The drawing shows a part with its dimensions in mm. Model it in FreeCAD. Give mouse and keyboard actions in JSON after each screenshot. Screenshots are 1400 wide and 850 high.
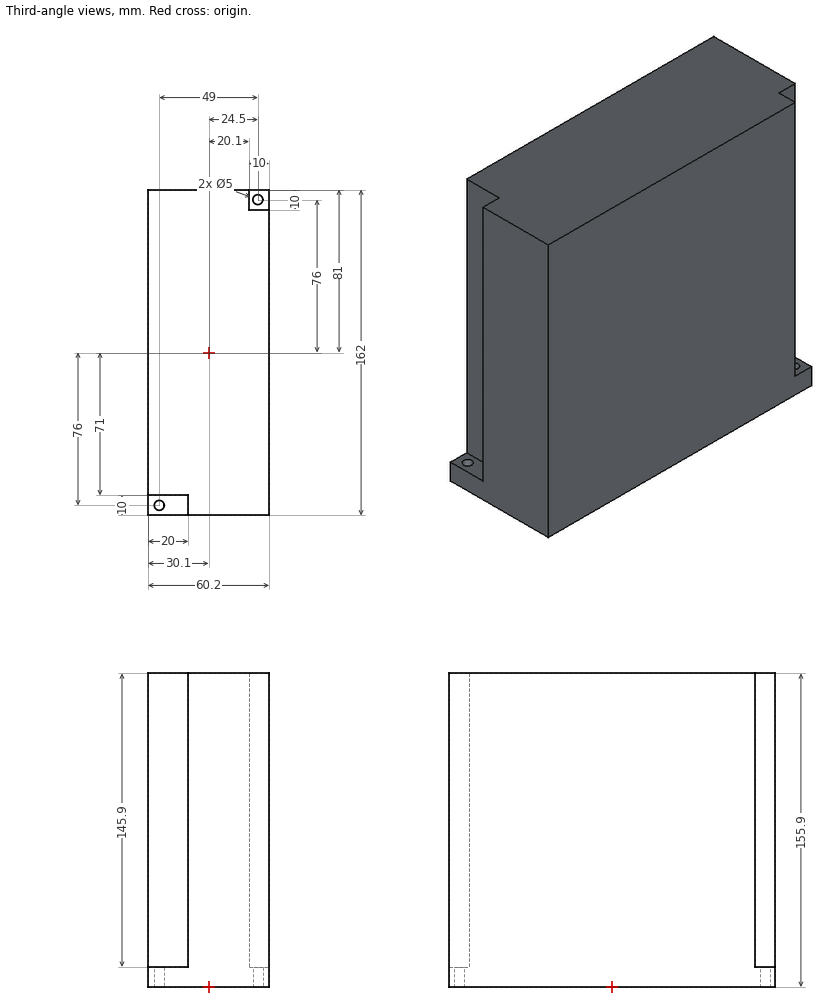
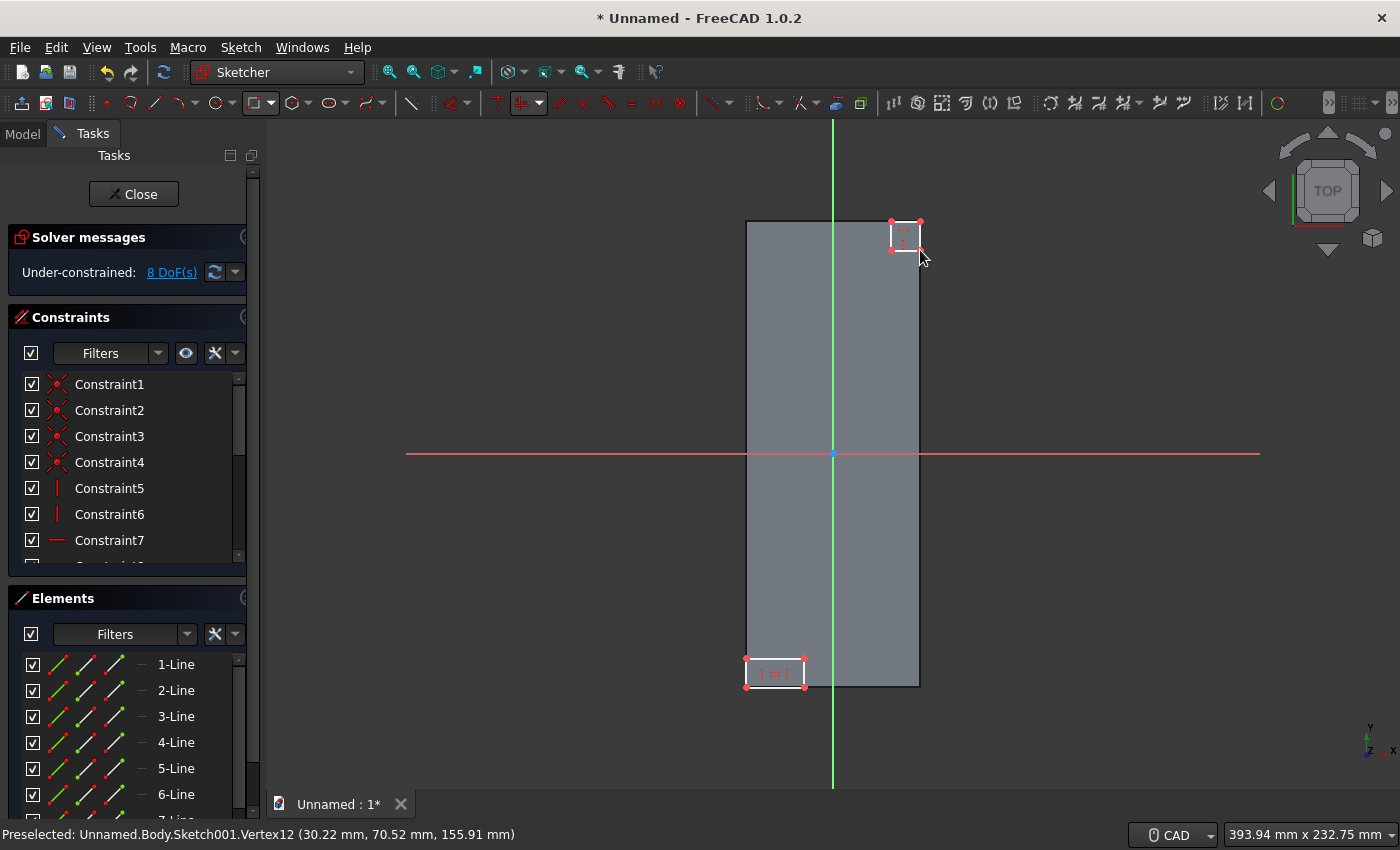
{"action": "key", "text": "d"}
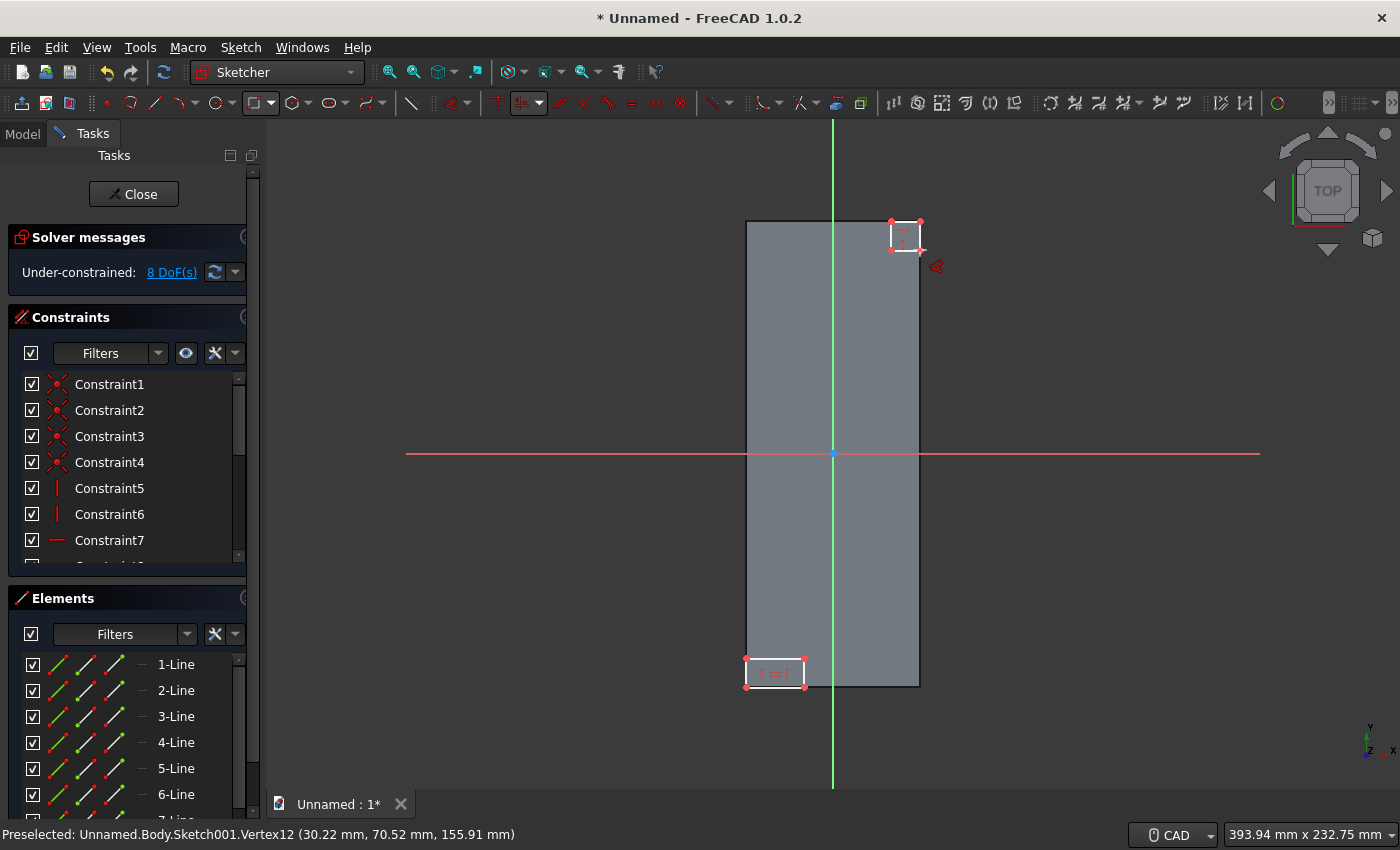
{"action": "scroll", "coordinate": [746, 671], "scroll_direction": "up", "scroll_amount": 2}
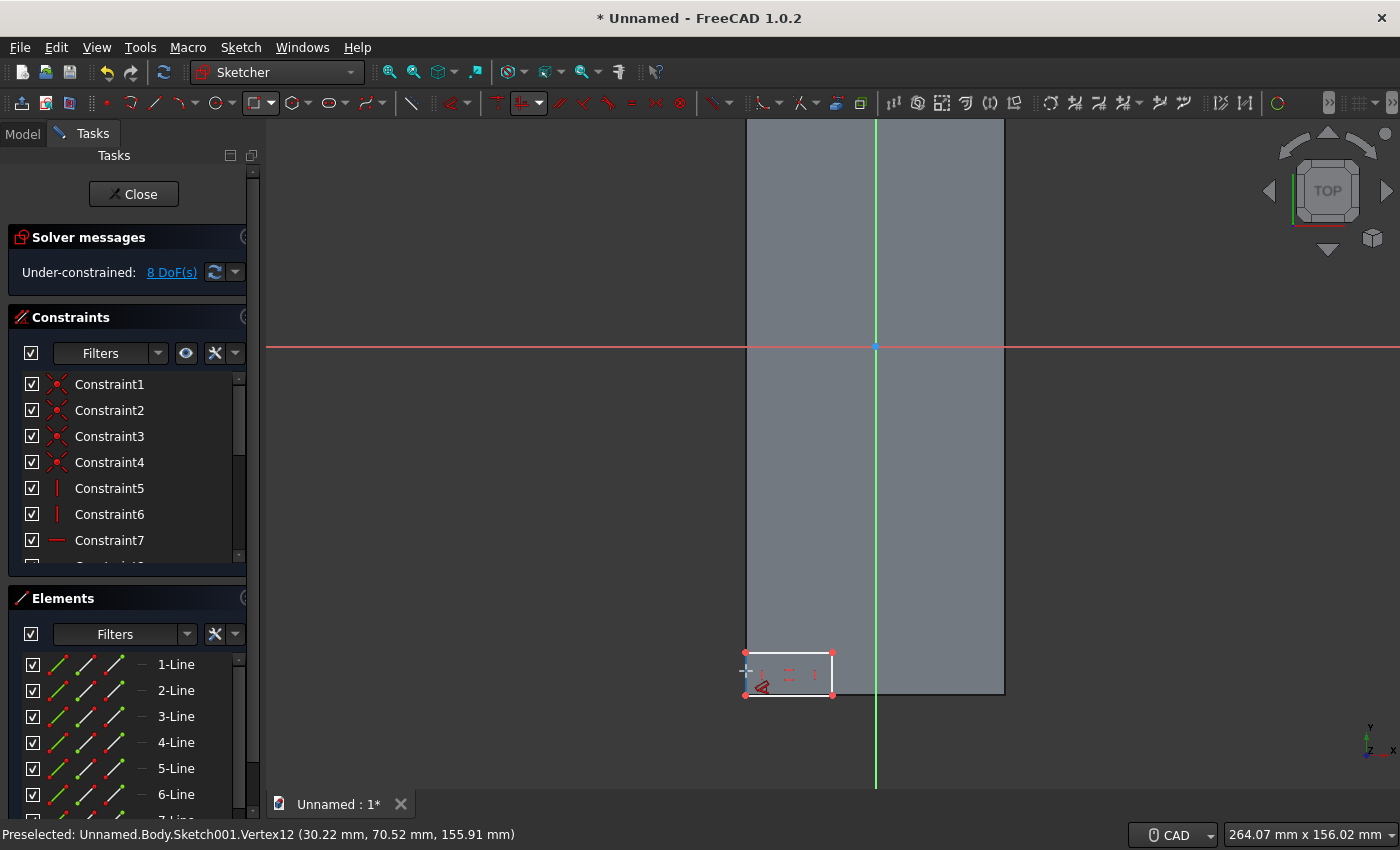
{"action": "left_click", "coordinate": [746, 670]}
{"action": "left_click", "coordinate": [712, 674]}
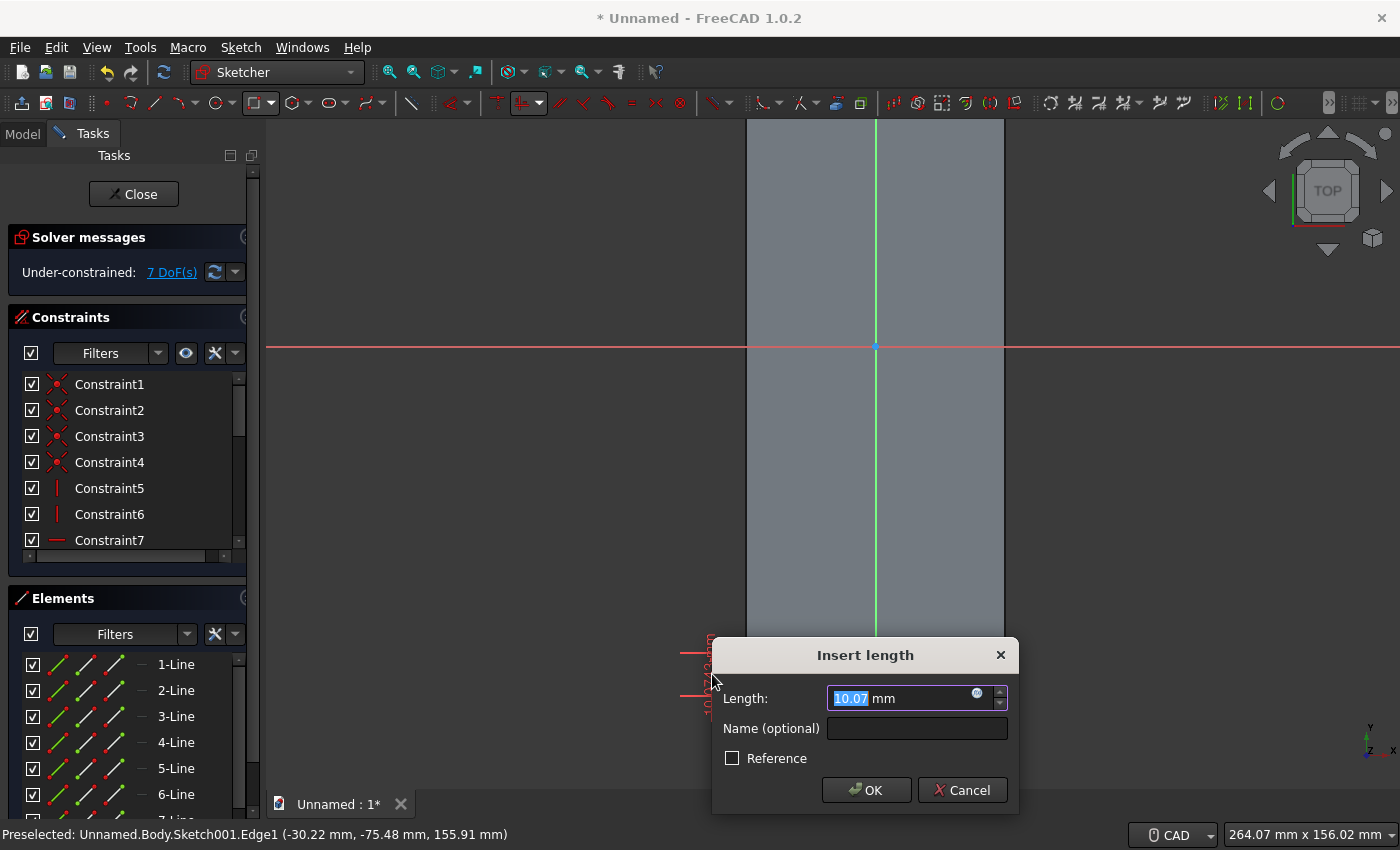
{"action": "type", "text": "10"}
{"action": "key", "text": "Return"}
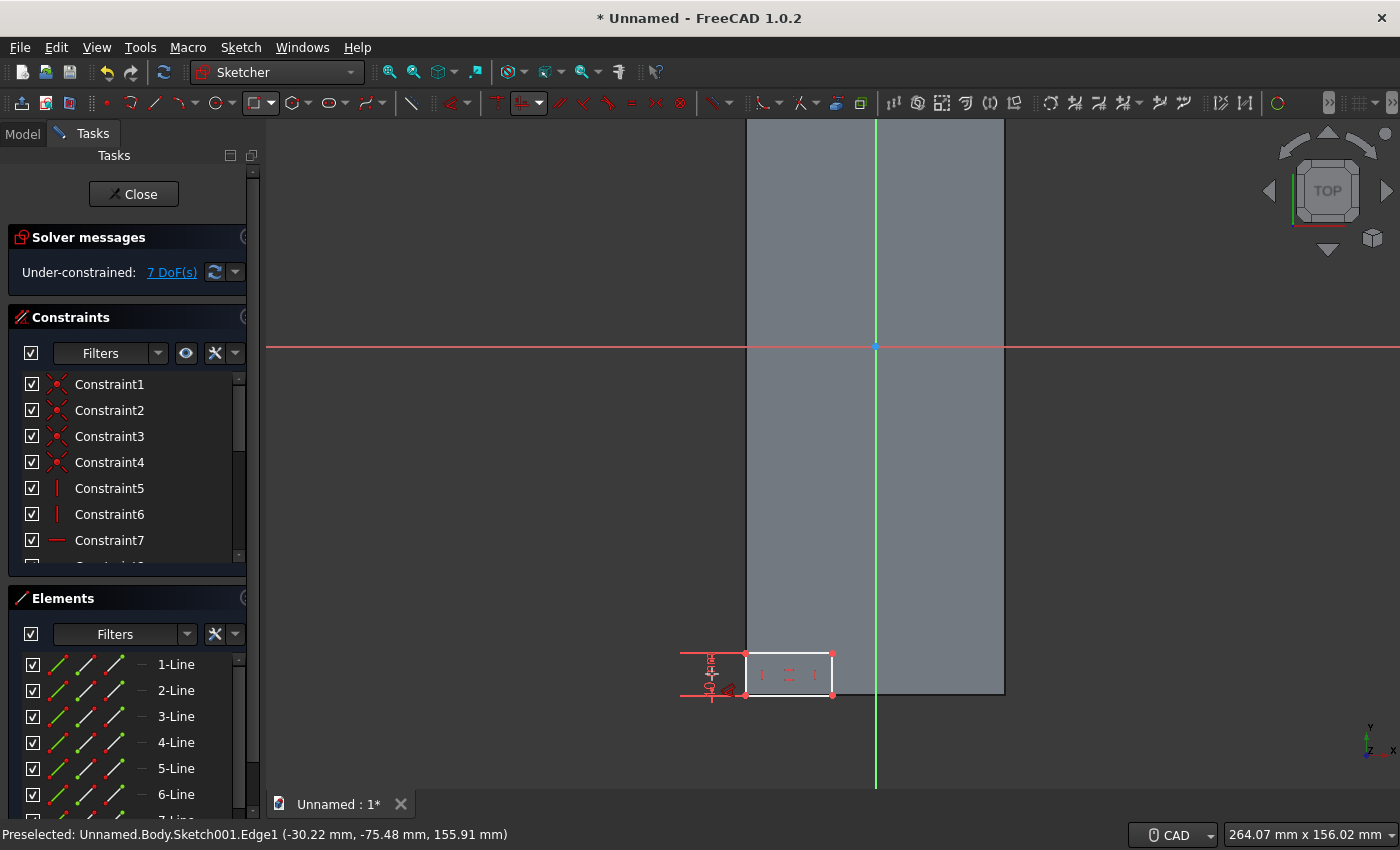
{"action": "left_click", "coordinate": [772, 696]}
{"action": "left_click", "coordinate": [789, 730]}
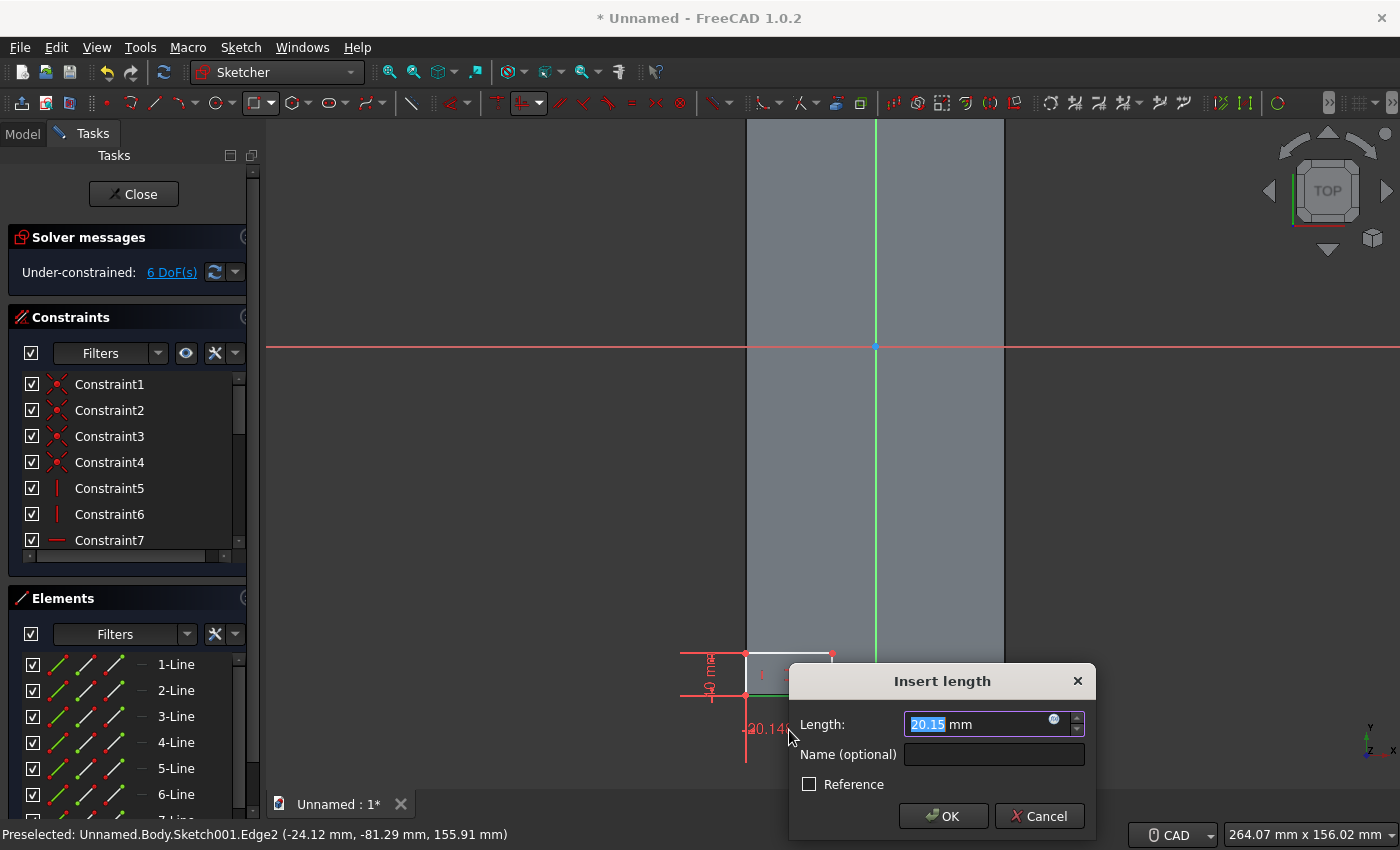
{"action": "type", "text": "20"}
{"action": "key", "text": "Return"}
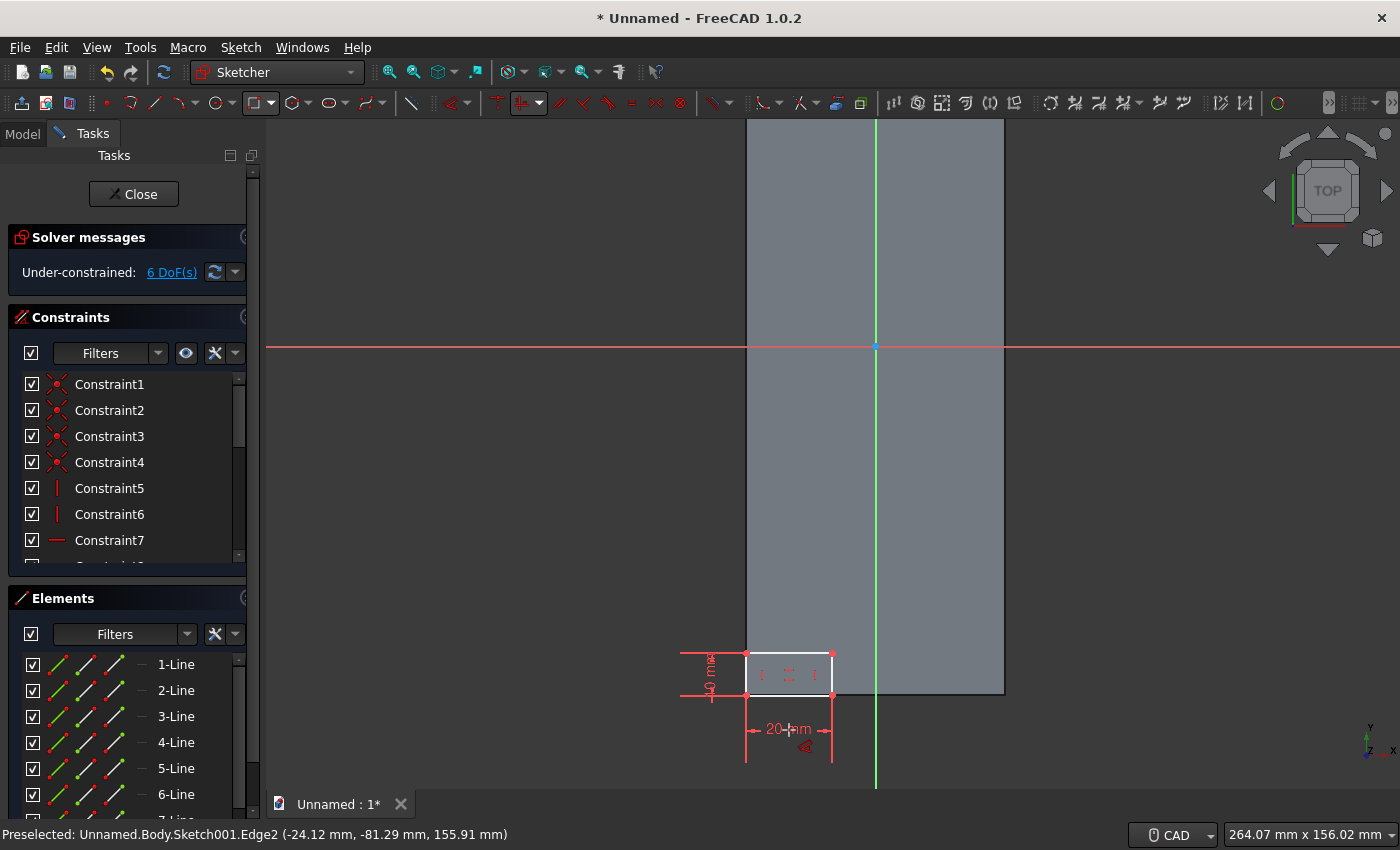
{"action": "scroll", "coordinate": [539, 672], "scroll_direction": "down", "scroll_amount": 2}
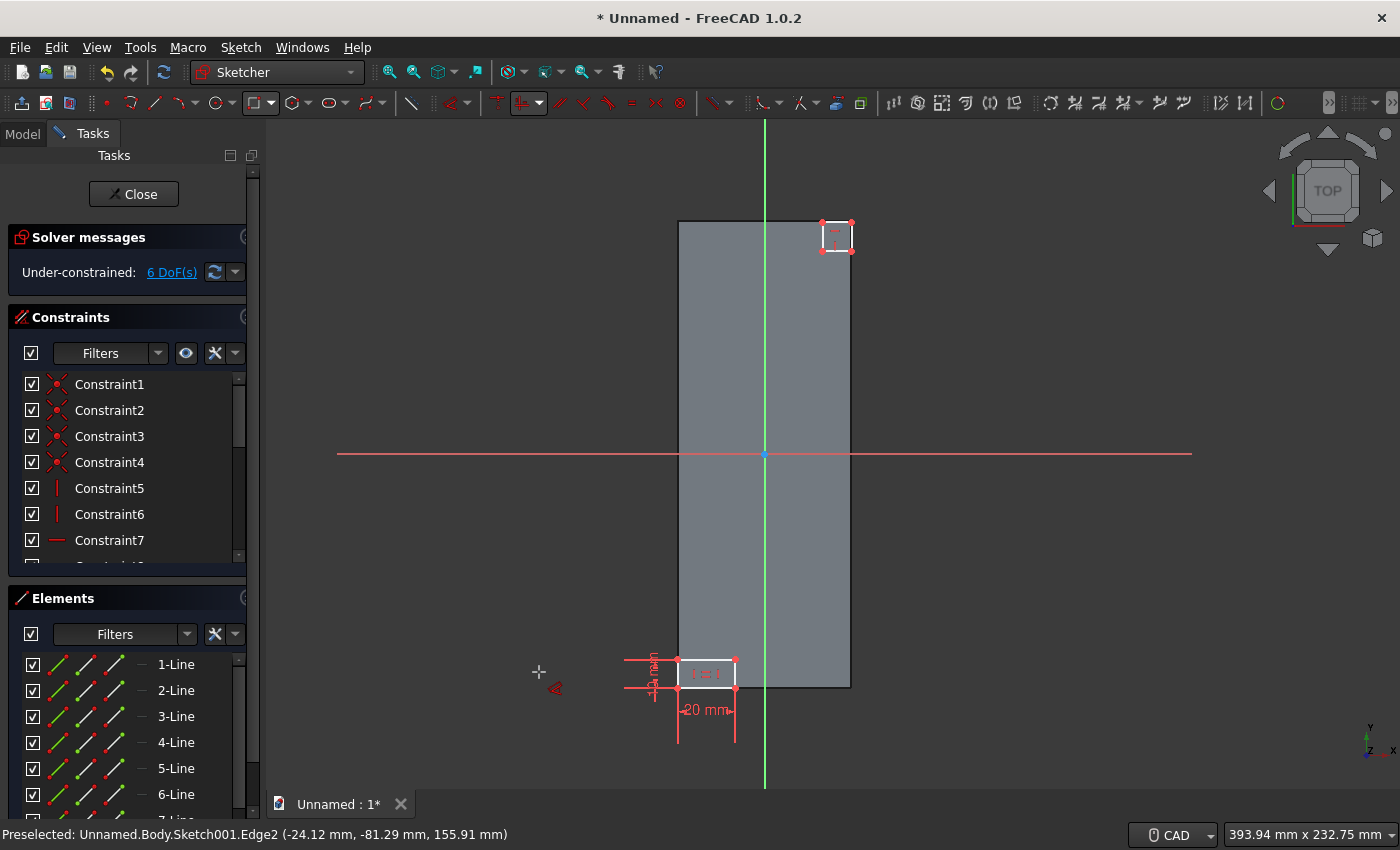
{"action": "scroll", "coordinate": [823, 231], "scroll_direction": "up", "scroll_amount": 3}